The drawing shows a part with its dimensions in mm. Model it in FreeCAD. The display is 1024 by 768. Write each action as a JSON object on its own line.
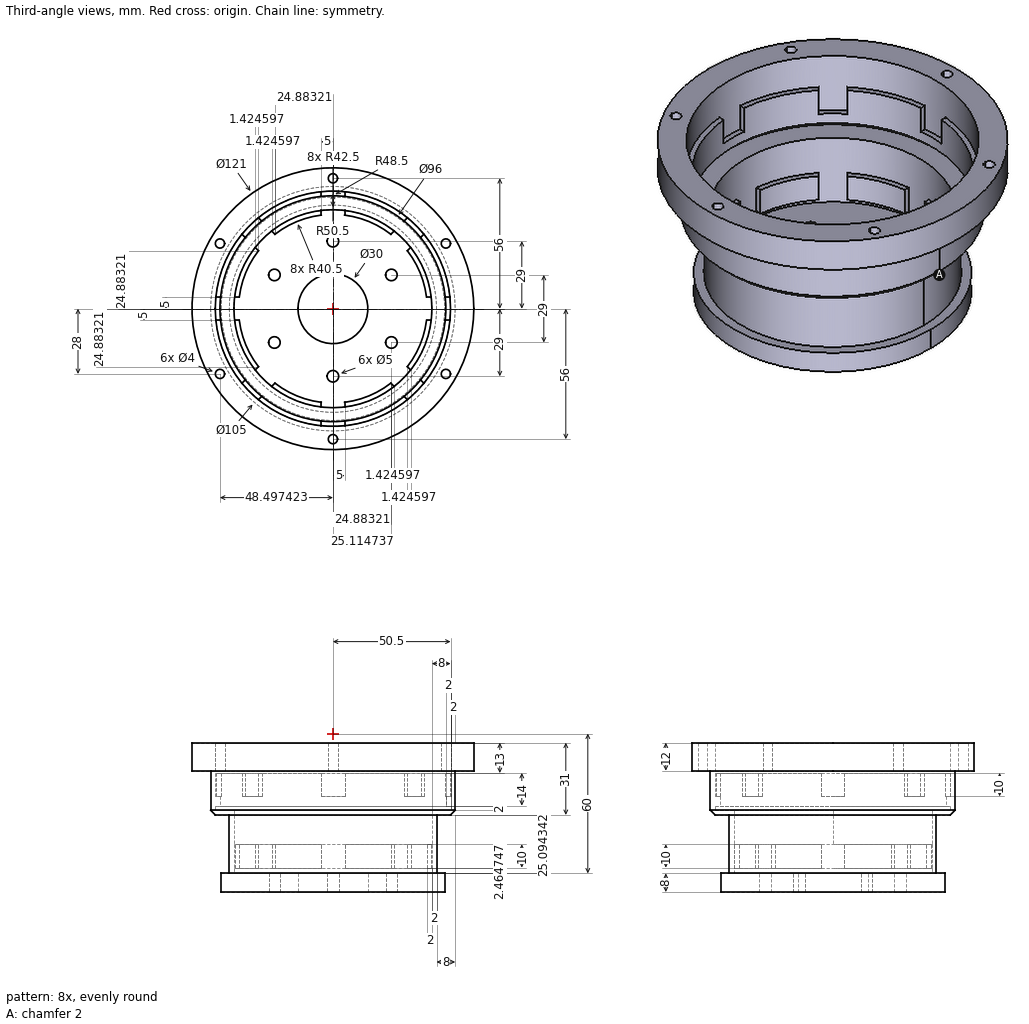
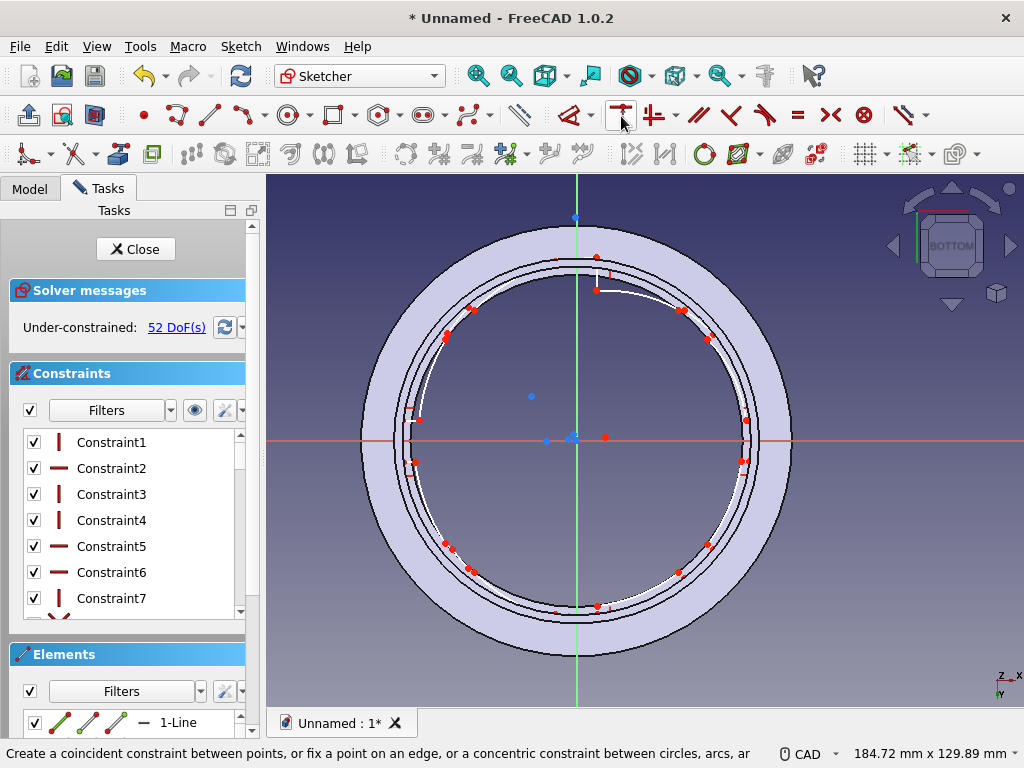
{"action": "left_click", "coordinate": [496, 591]}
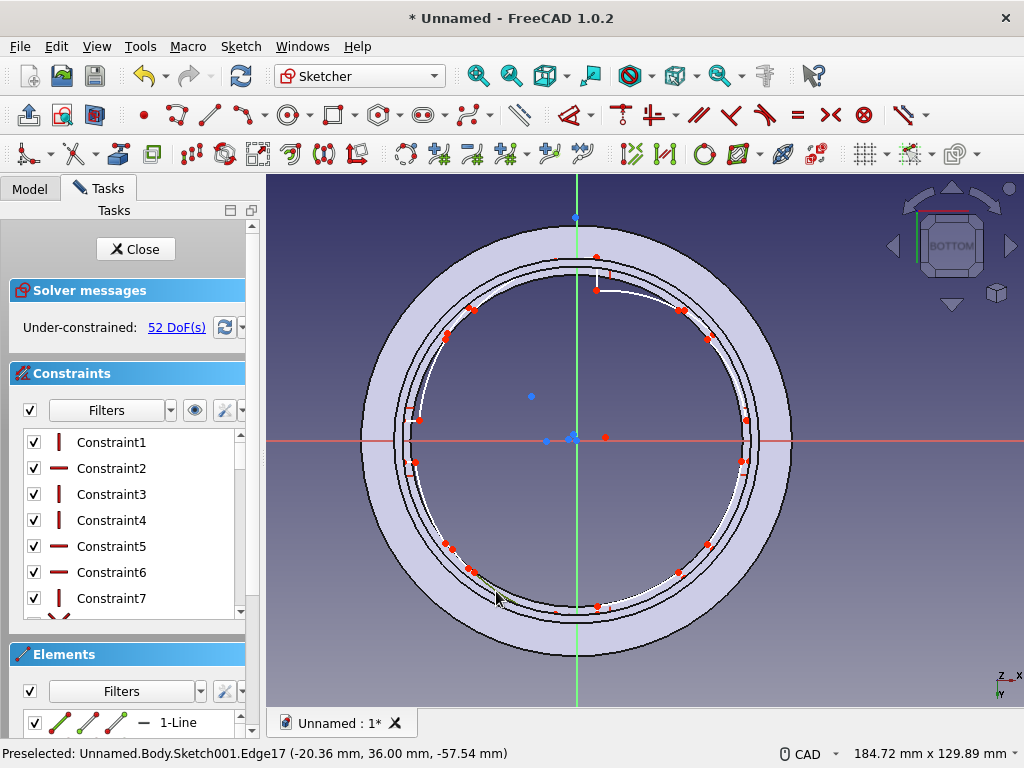
{"action": "left_click", "coordinate": [751, 441]}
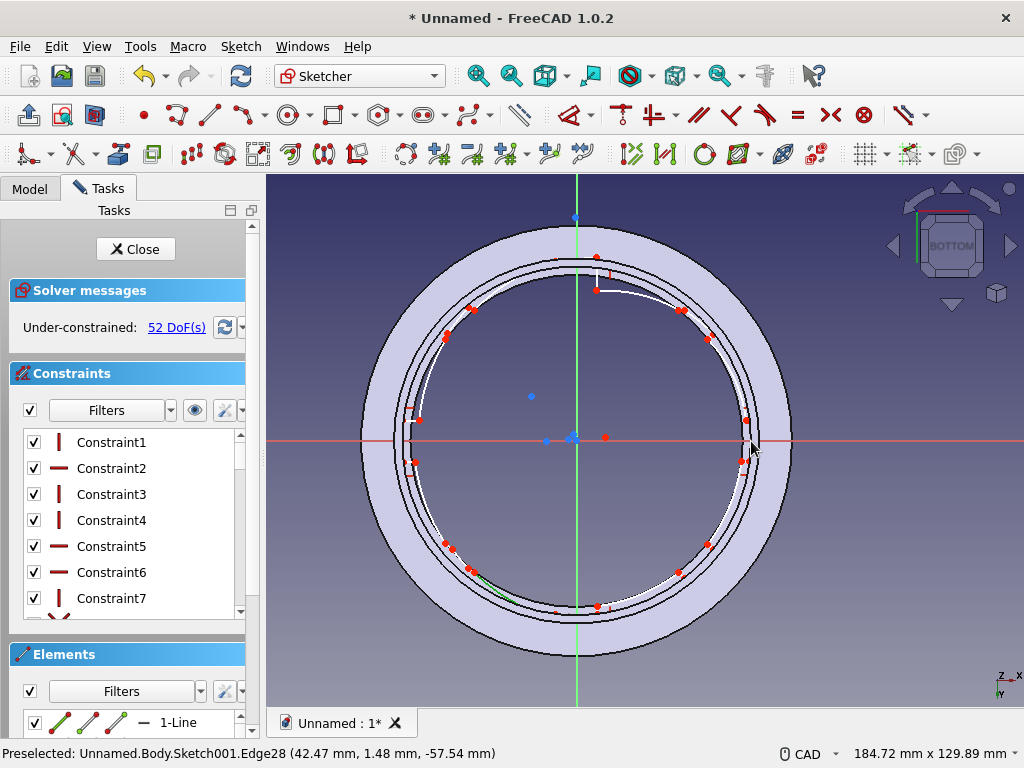
{"action": "key", "text": "c"}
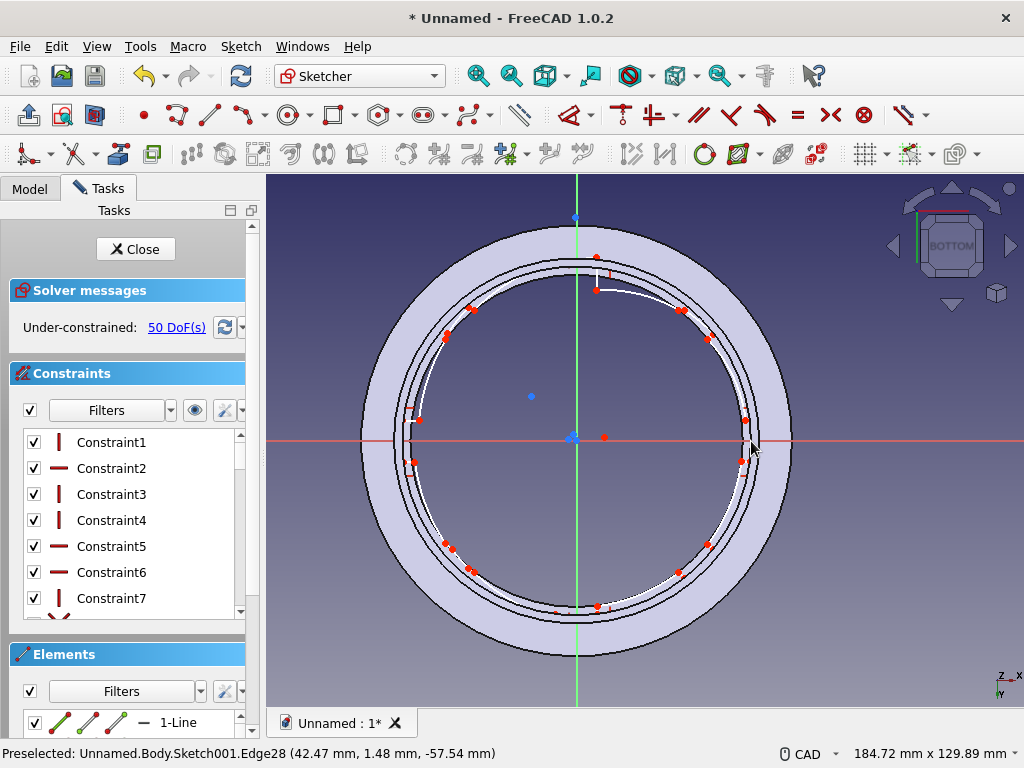
{"action": "left_click", "coordinate": [496, 591]}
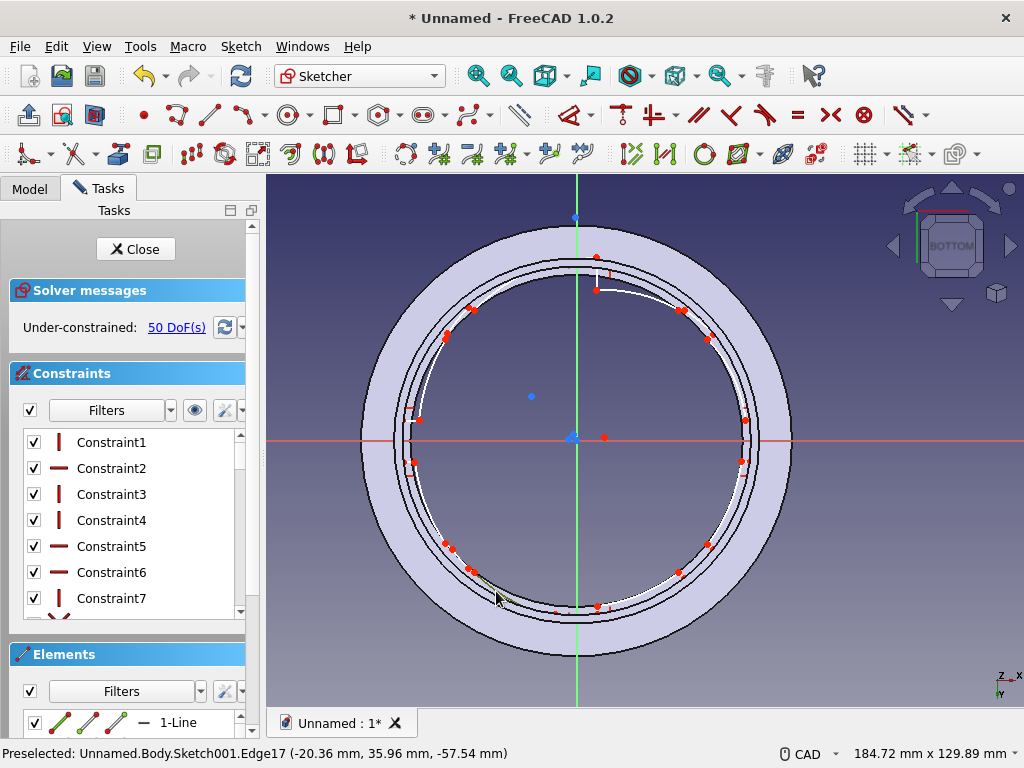
{"action": "left_click", "coordinate": [722, 522]}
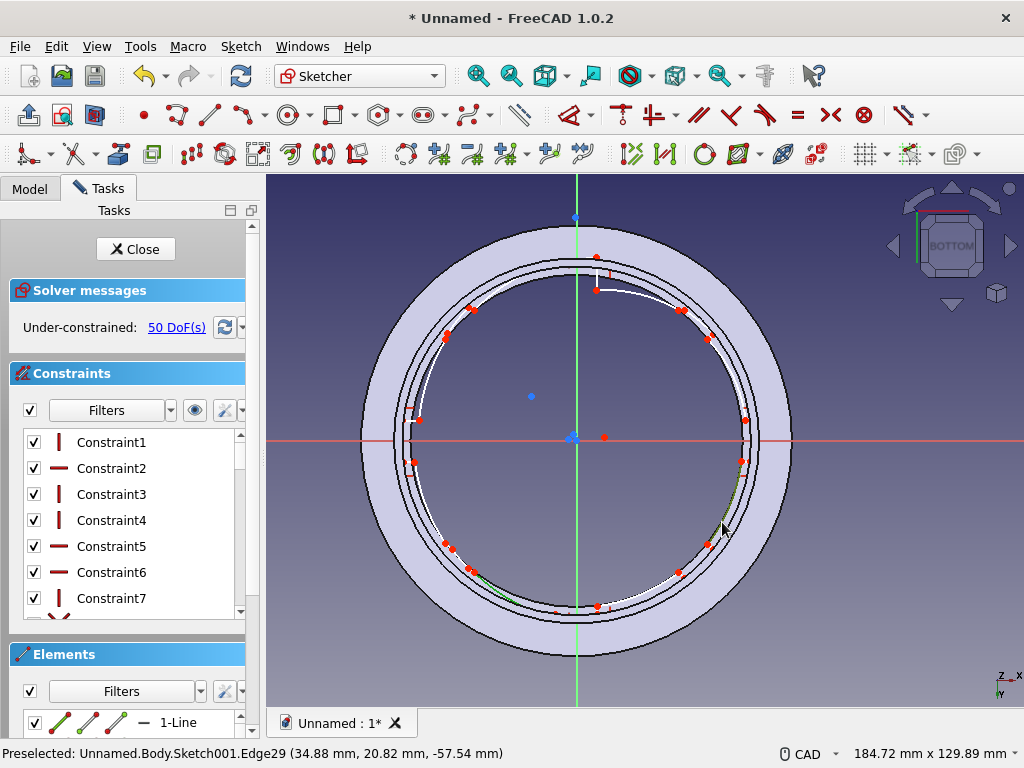
{"action": "key", "text": "c"}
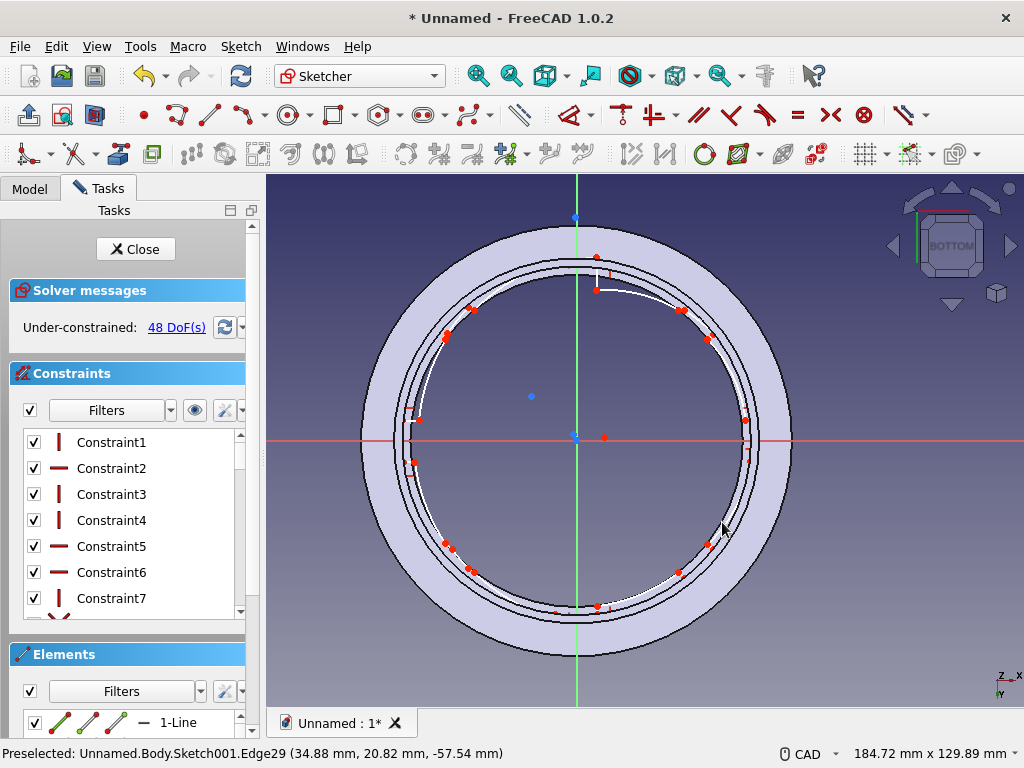
{"action": "left_click", "coordinate": [496, 591]}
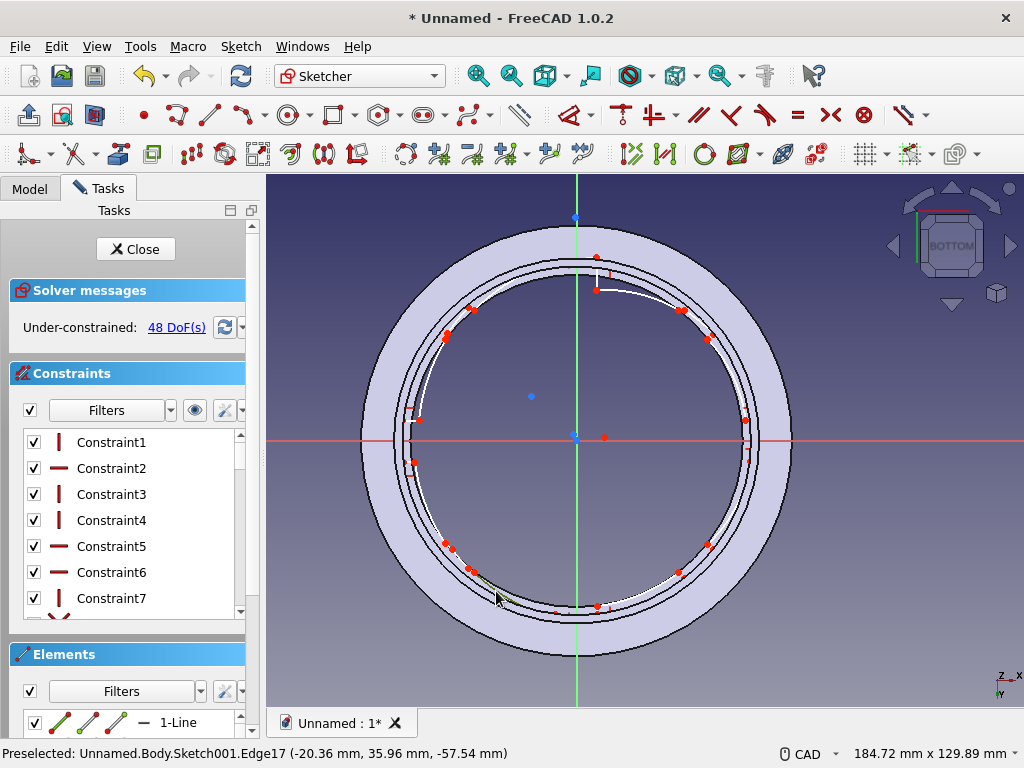
{"action": "left_click", "coordinate": [694, 570]}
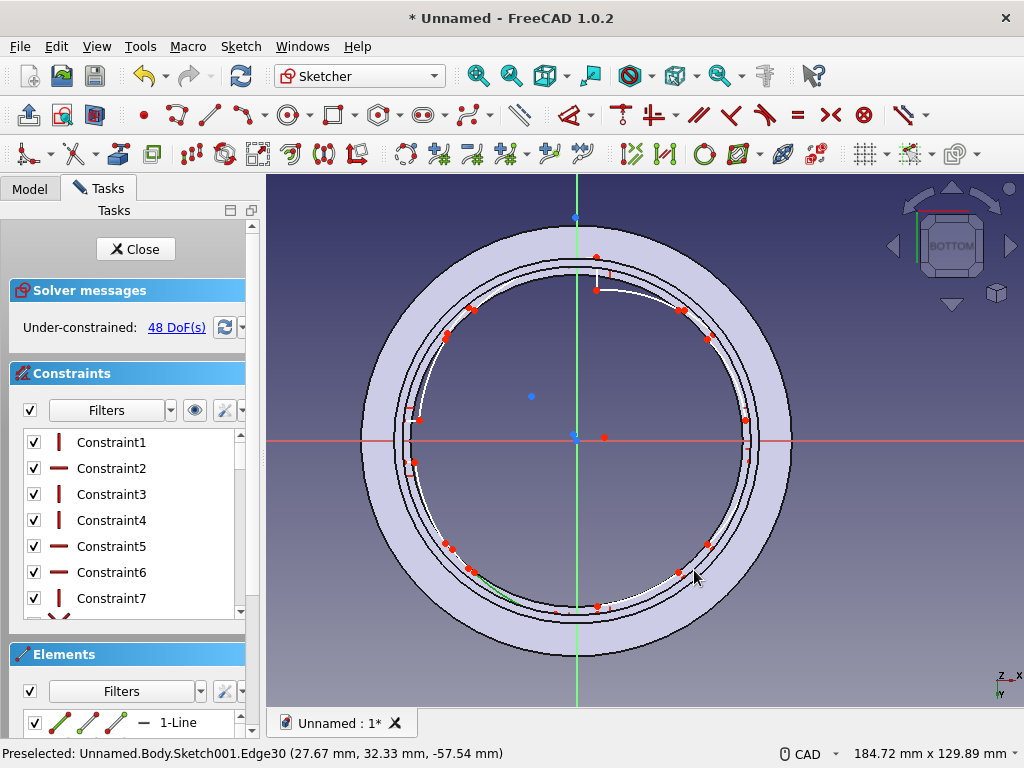
{"action": "key", "text": "c"}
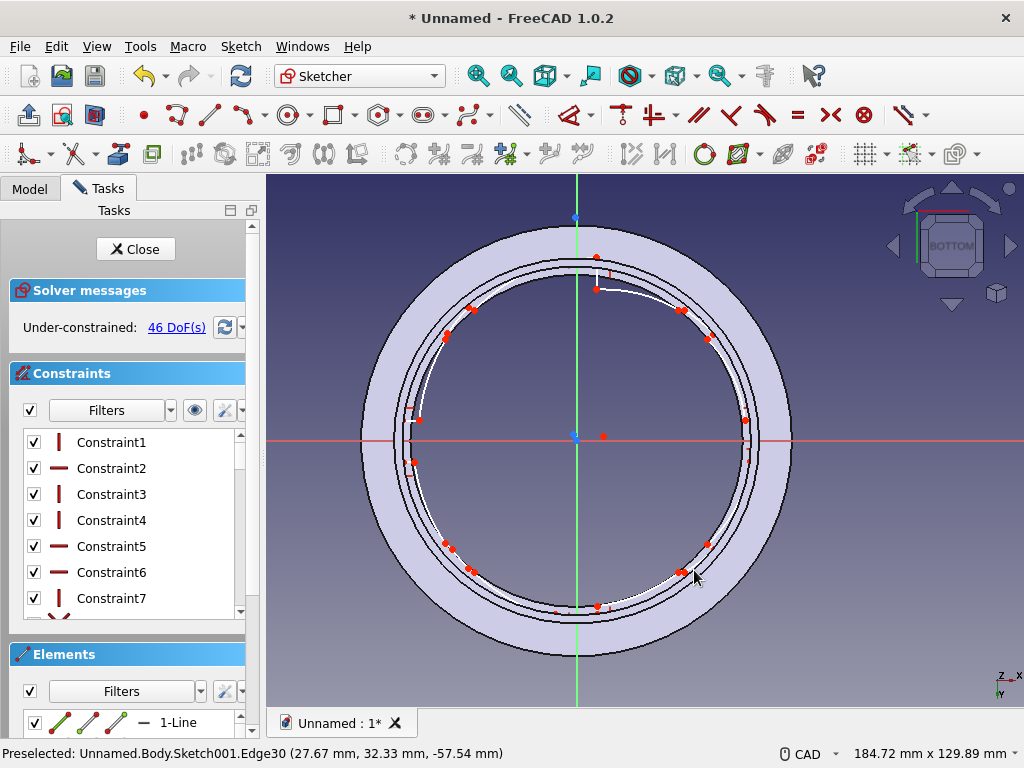
{"action": "left_click", "coordinate": [496, 590]}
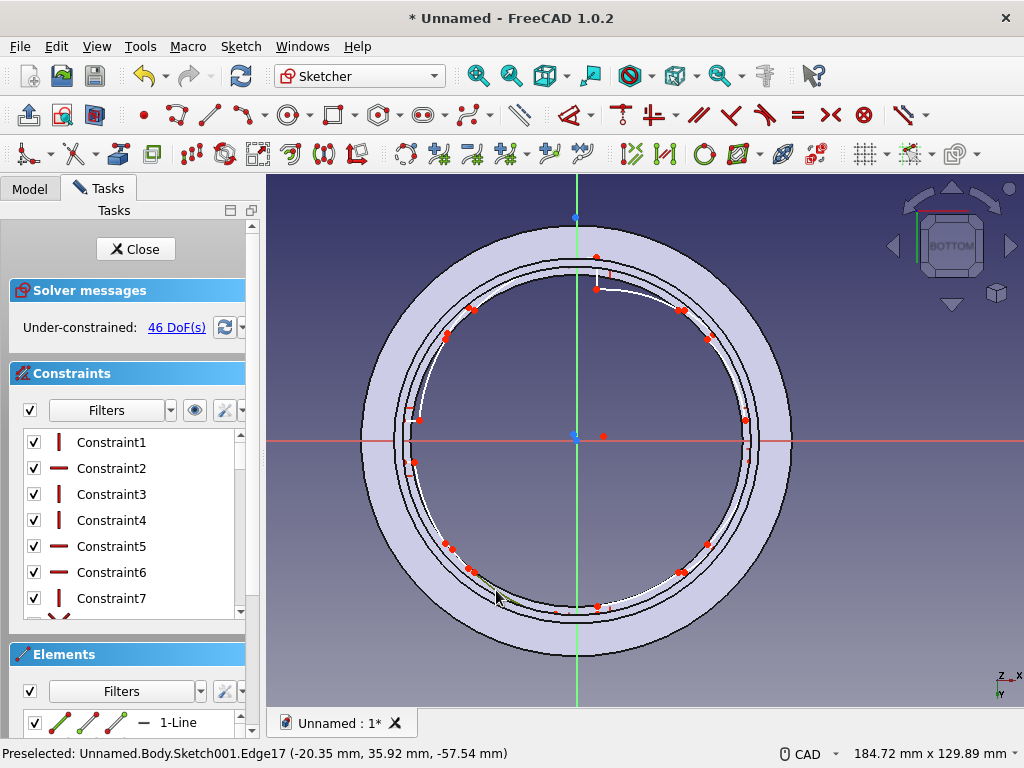
{"action": "left_click", "coordinate": [623, 601]}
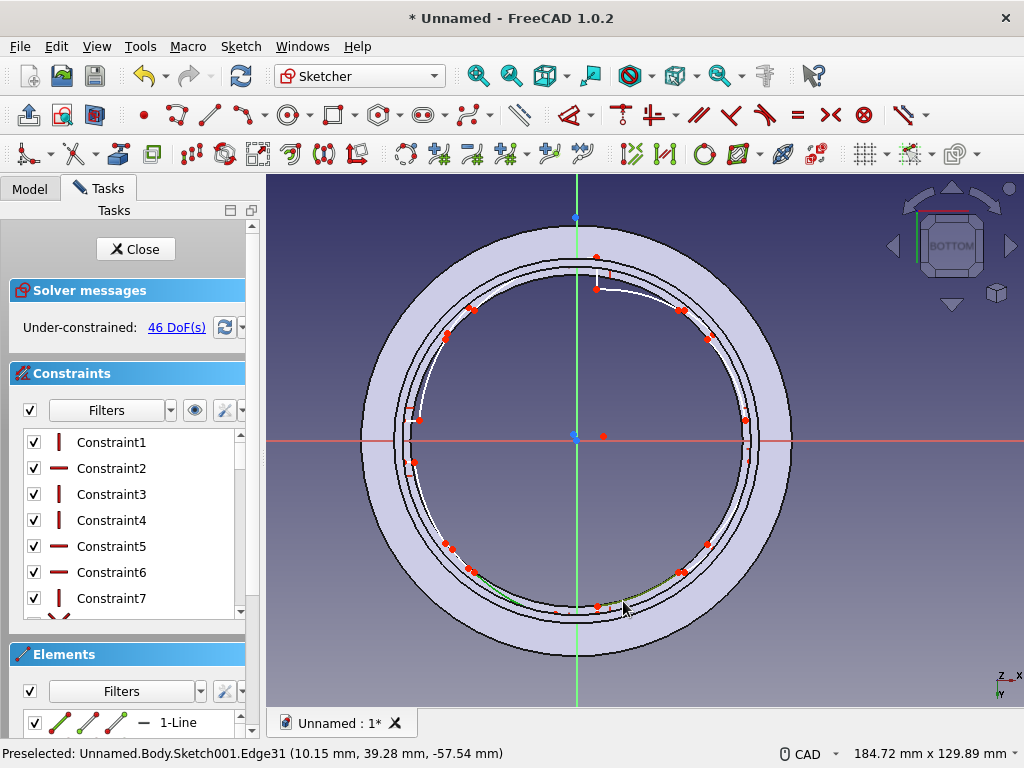
{"action": "key", "text": "c"}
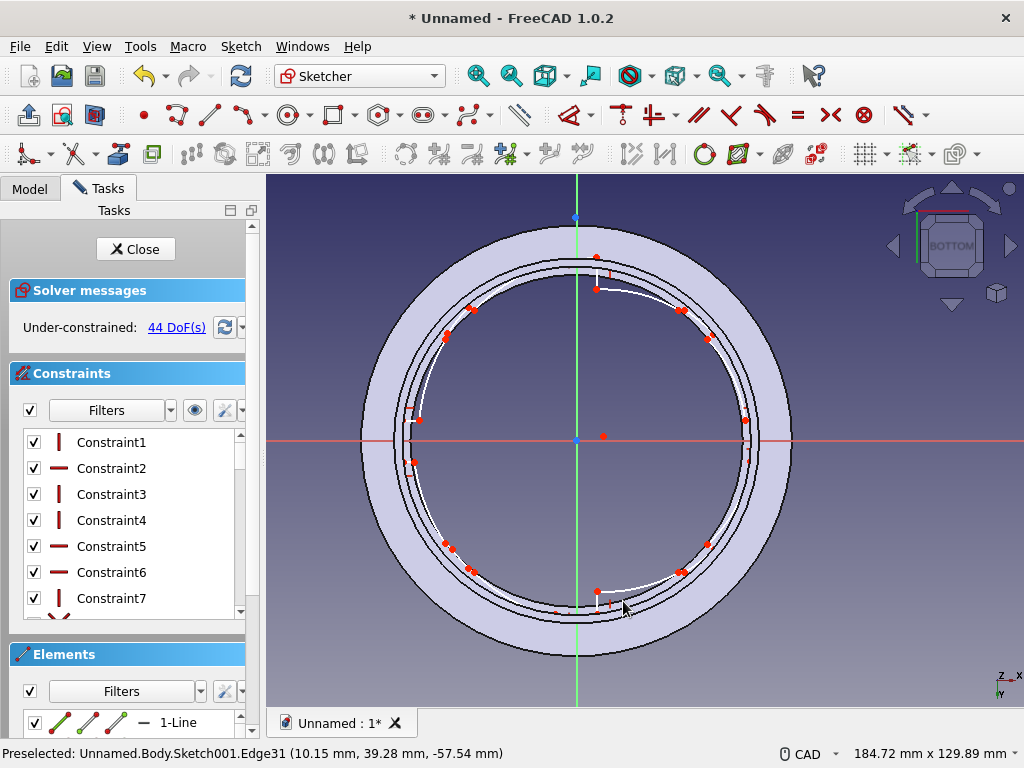
{"action": "left_click", "coordinate": [496, 590]}